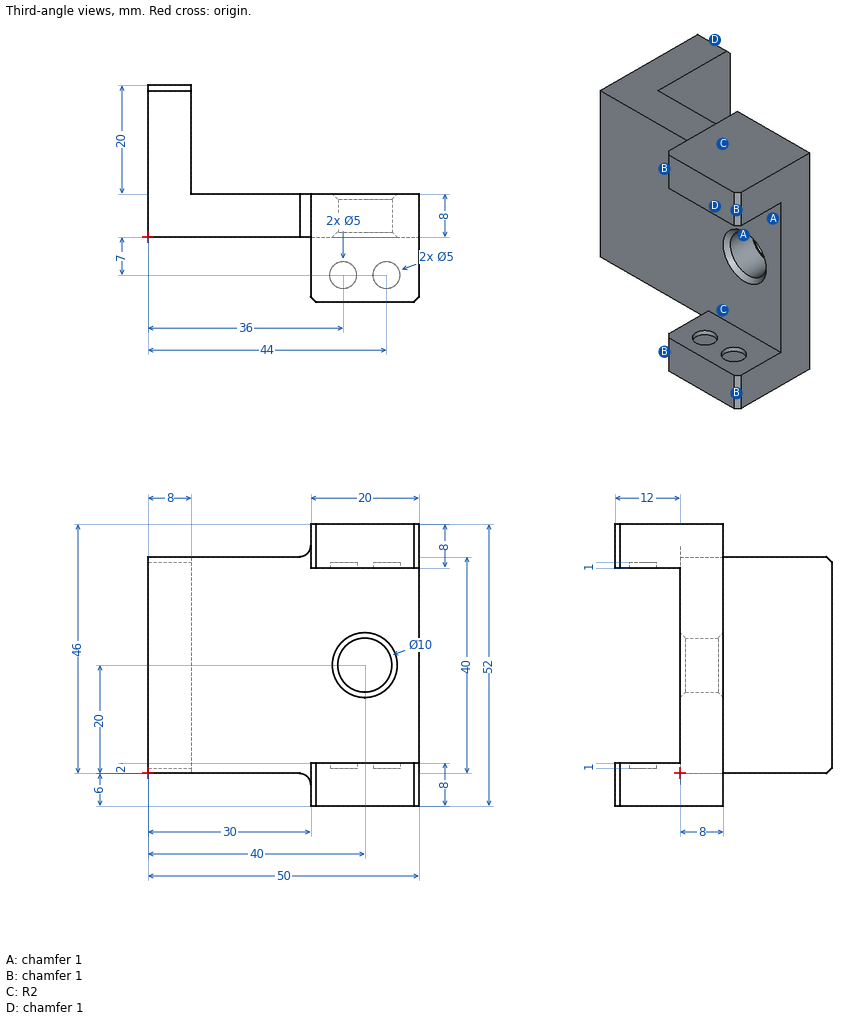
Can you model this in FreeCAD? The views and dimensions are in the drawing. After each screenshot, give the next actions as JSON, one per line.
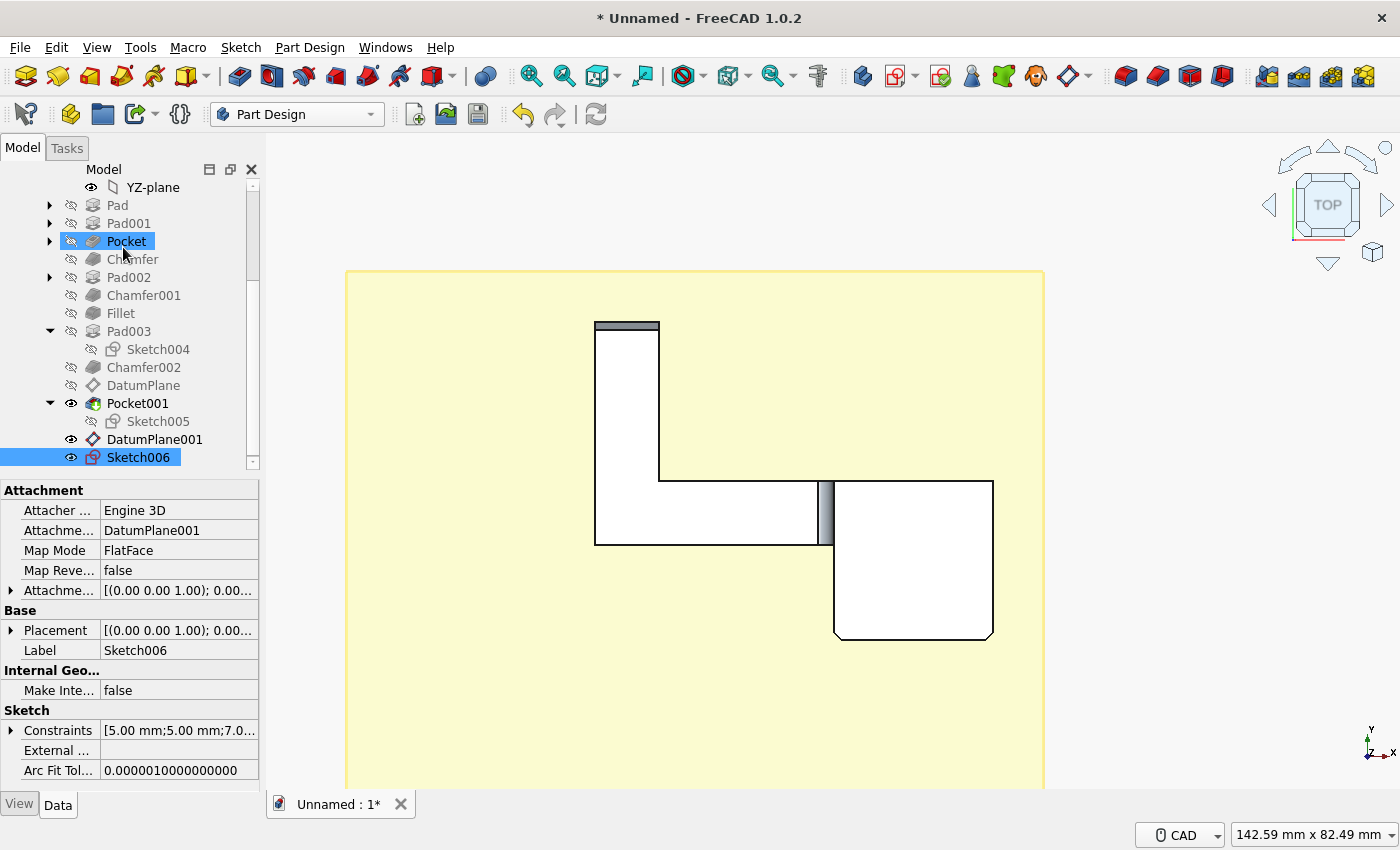
{"action": "left_click", "coordinate": [240, 76]}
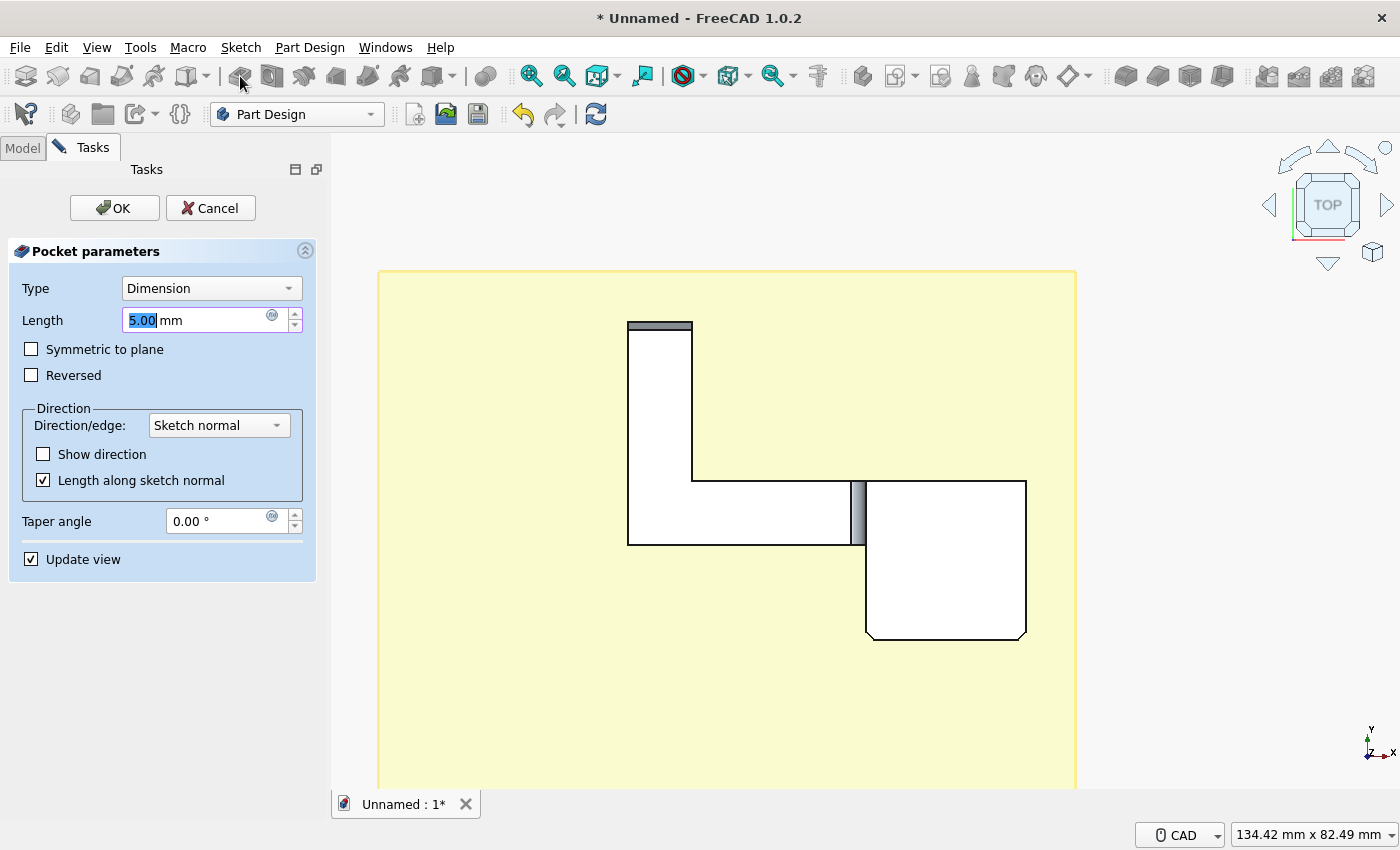
{"action": "type", "text": "1"}
{"action": "key", "text": "Tab"}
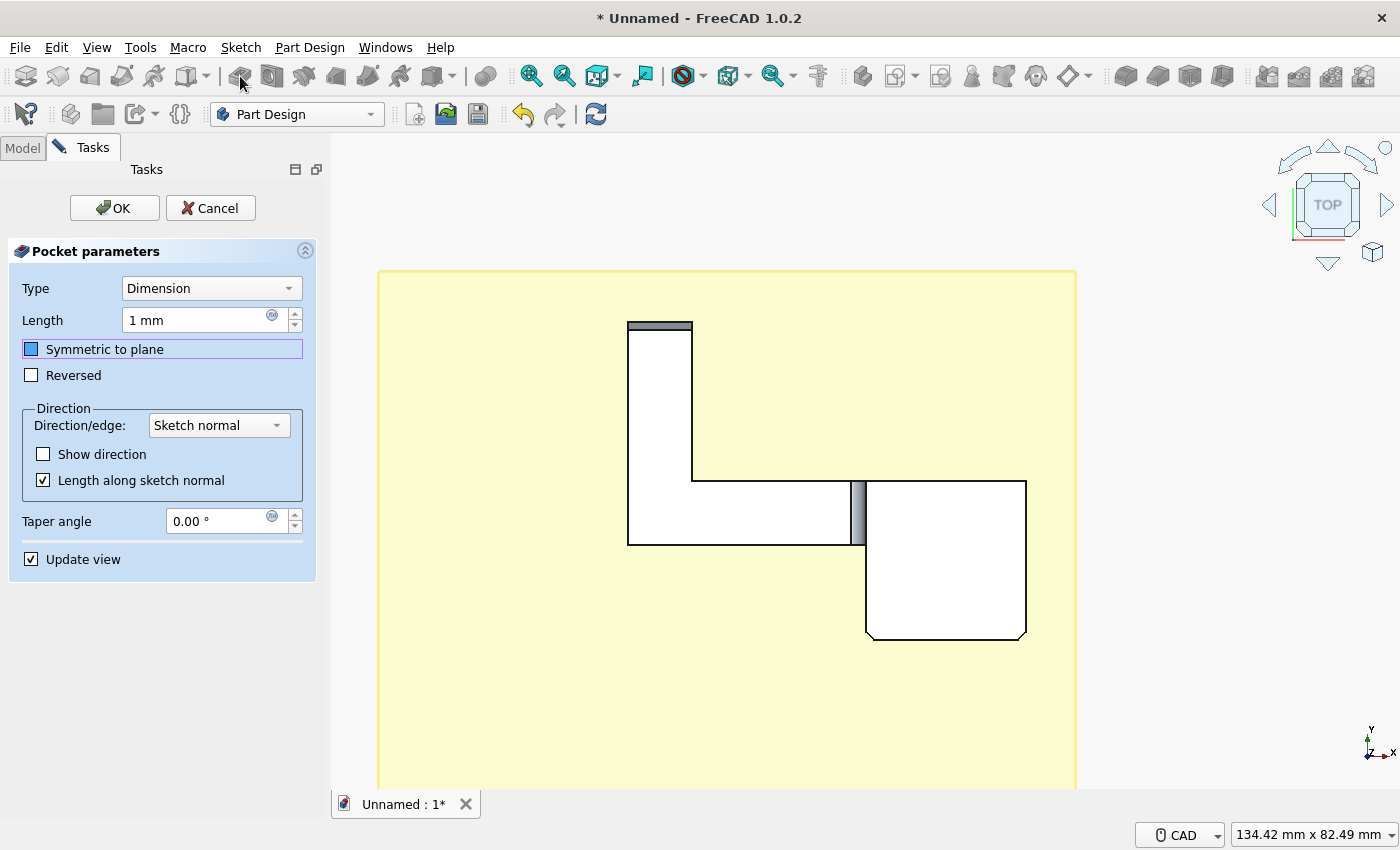
{"action": "left_click", "coordinate": [115, 208]}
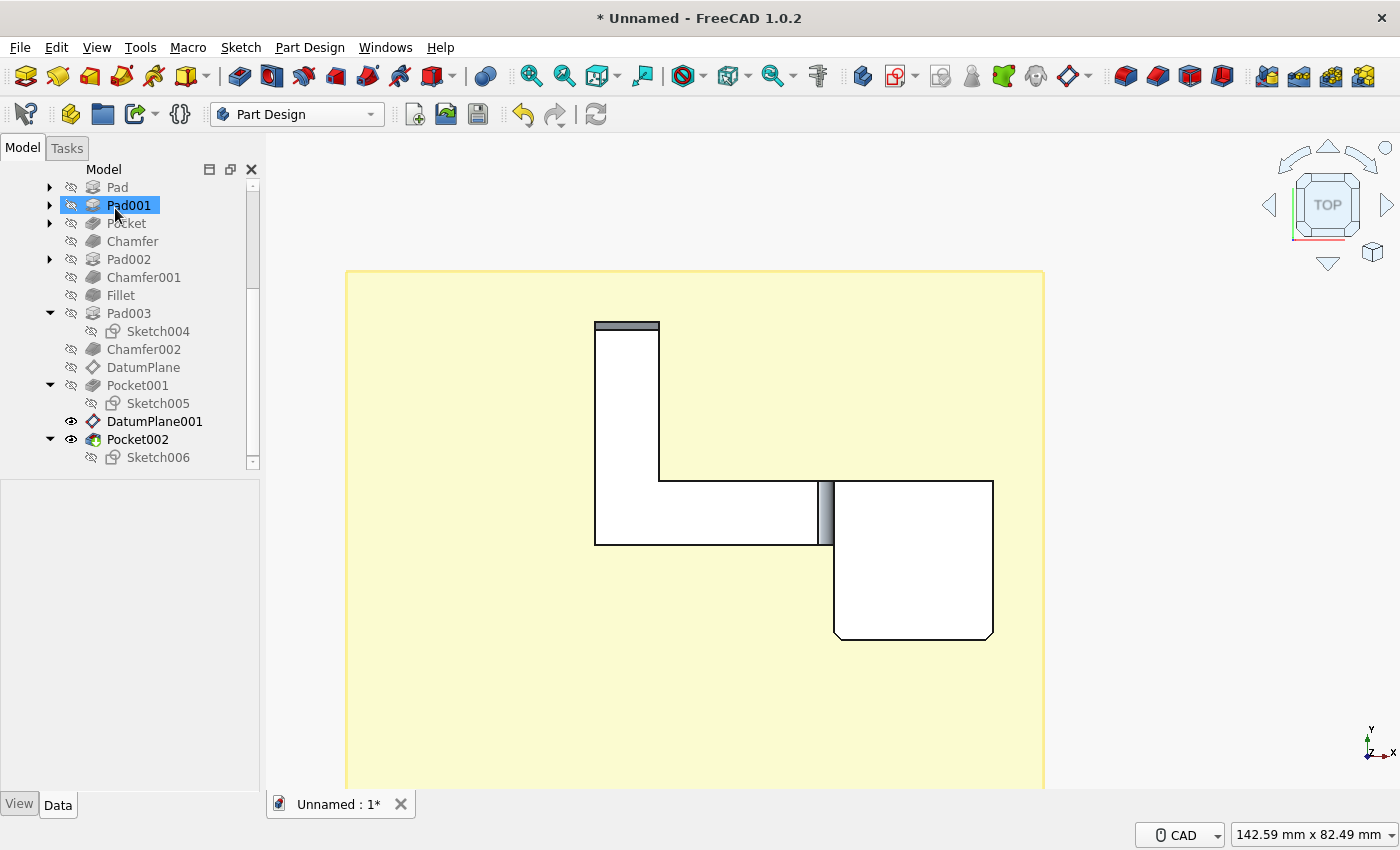
{"action": "left_click", "coordinate": [116, 421]}
{"action": "key", "text": "space"}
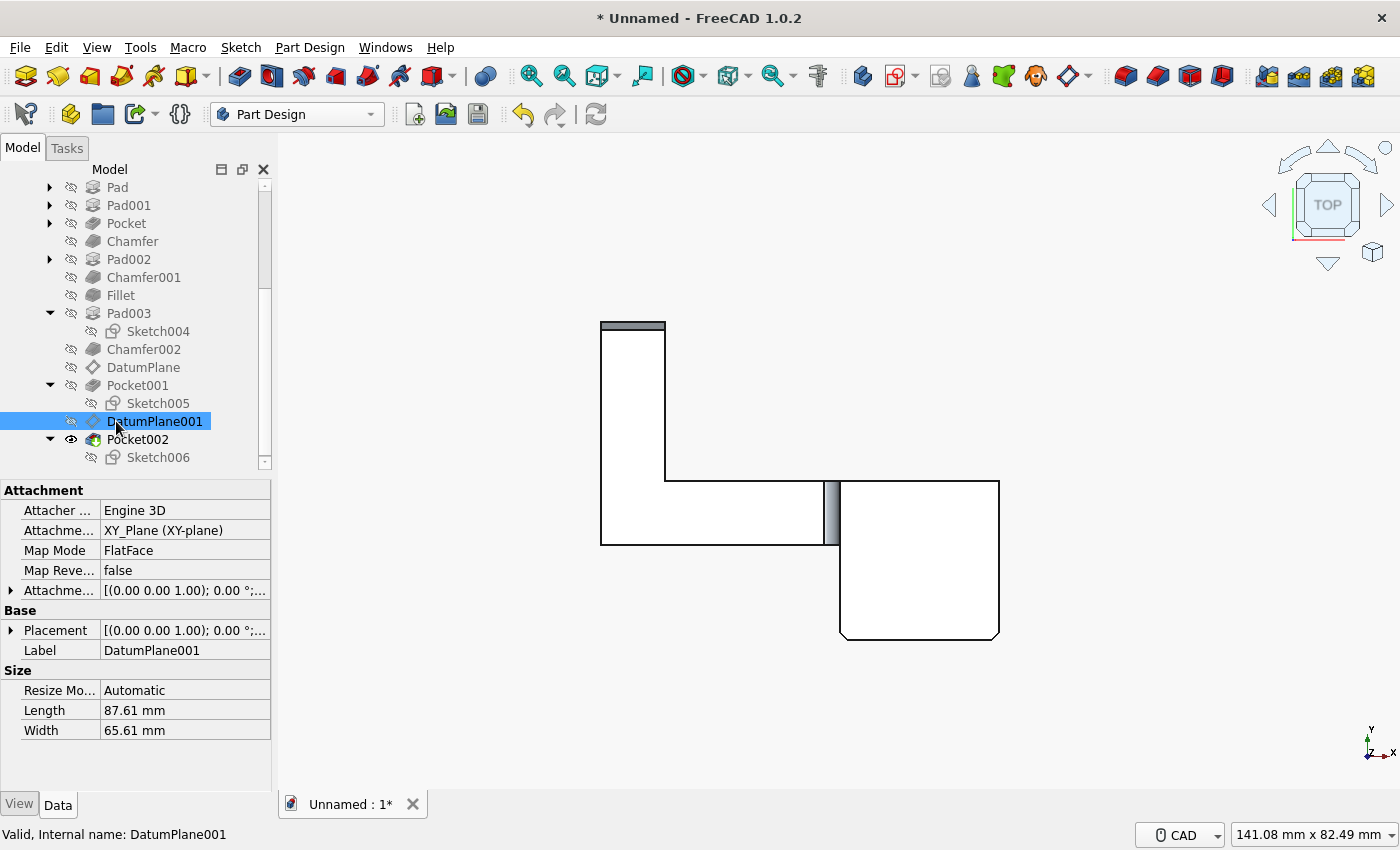
{"action": "key", "text": "0"}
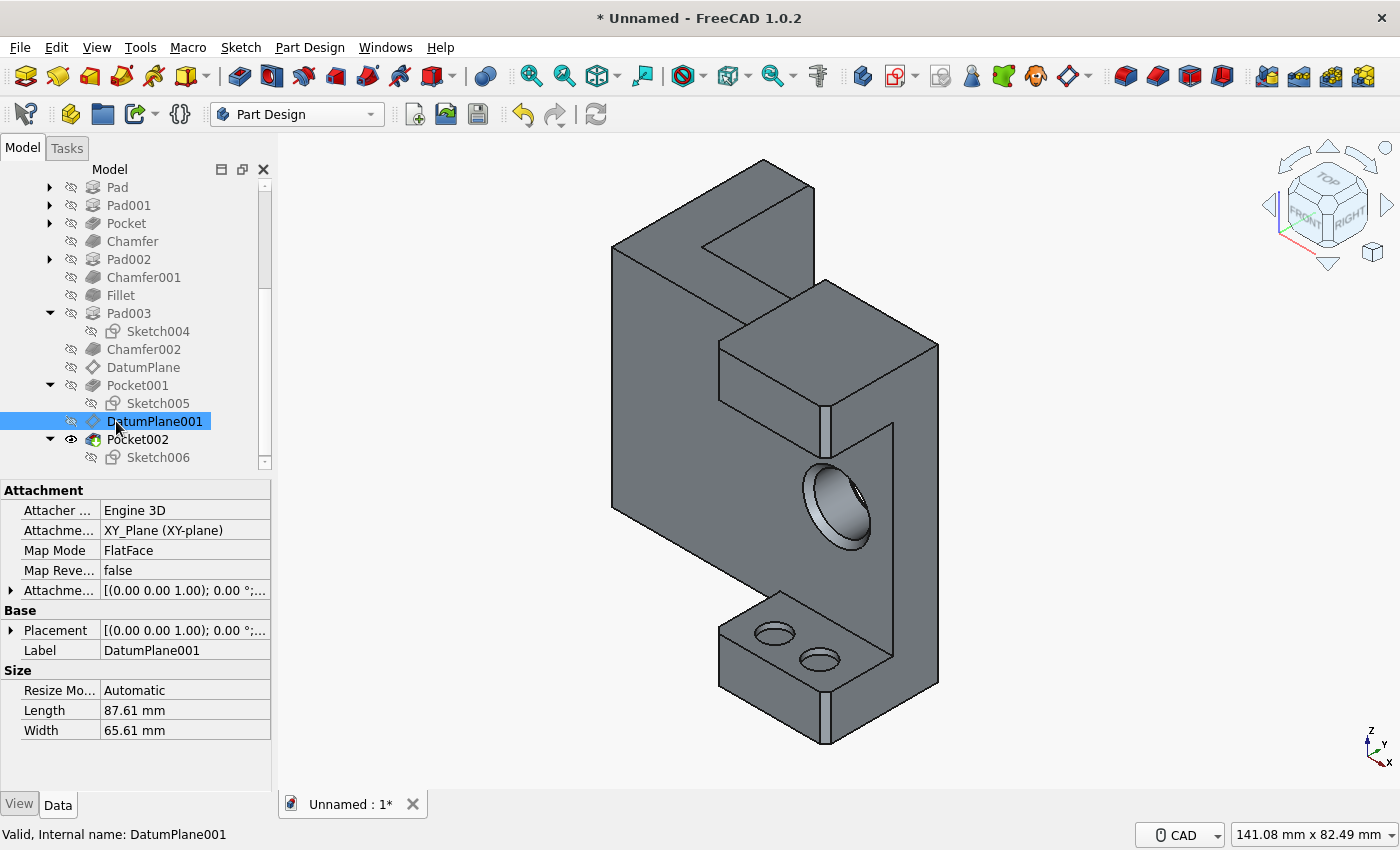
{"action": "key", "text": "v f"}